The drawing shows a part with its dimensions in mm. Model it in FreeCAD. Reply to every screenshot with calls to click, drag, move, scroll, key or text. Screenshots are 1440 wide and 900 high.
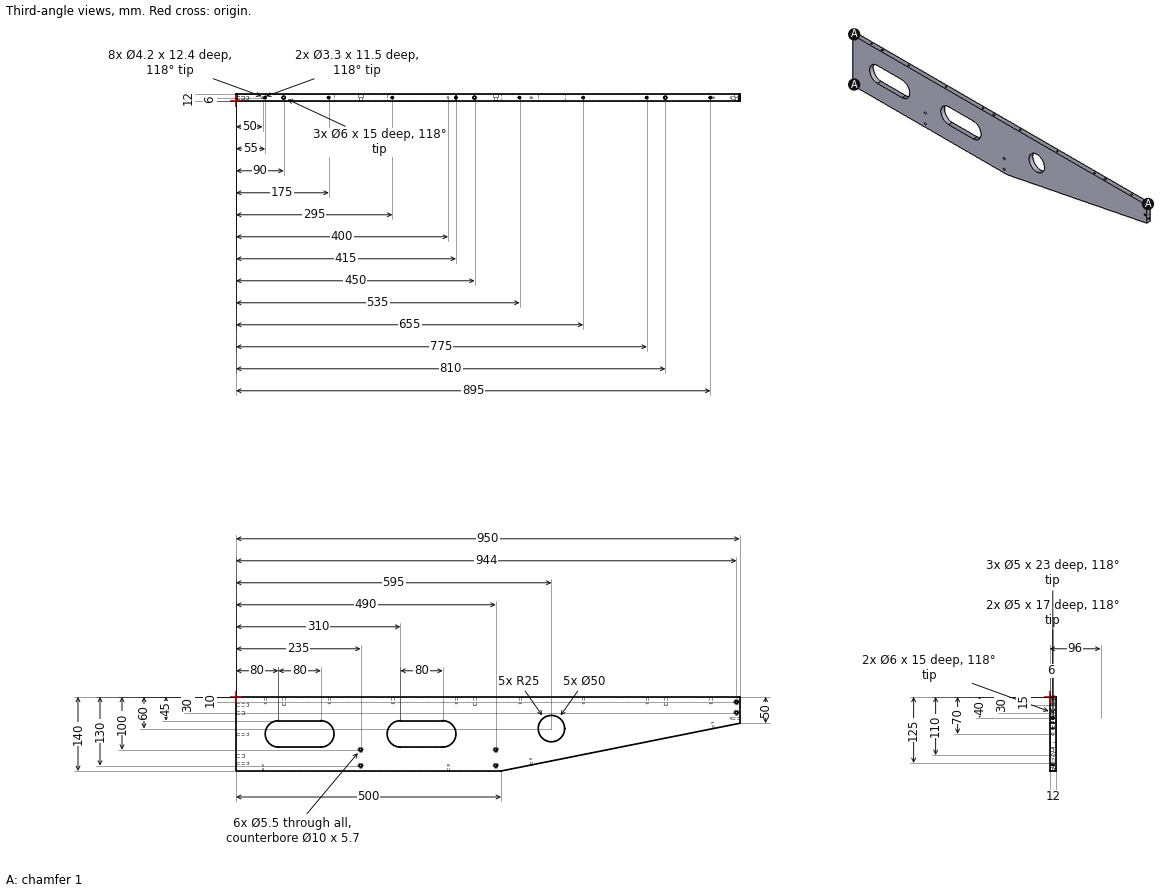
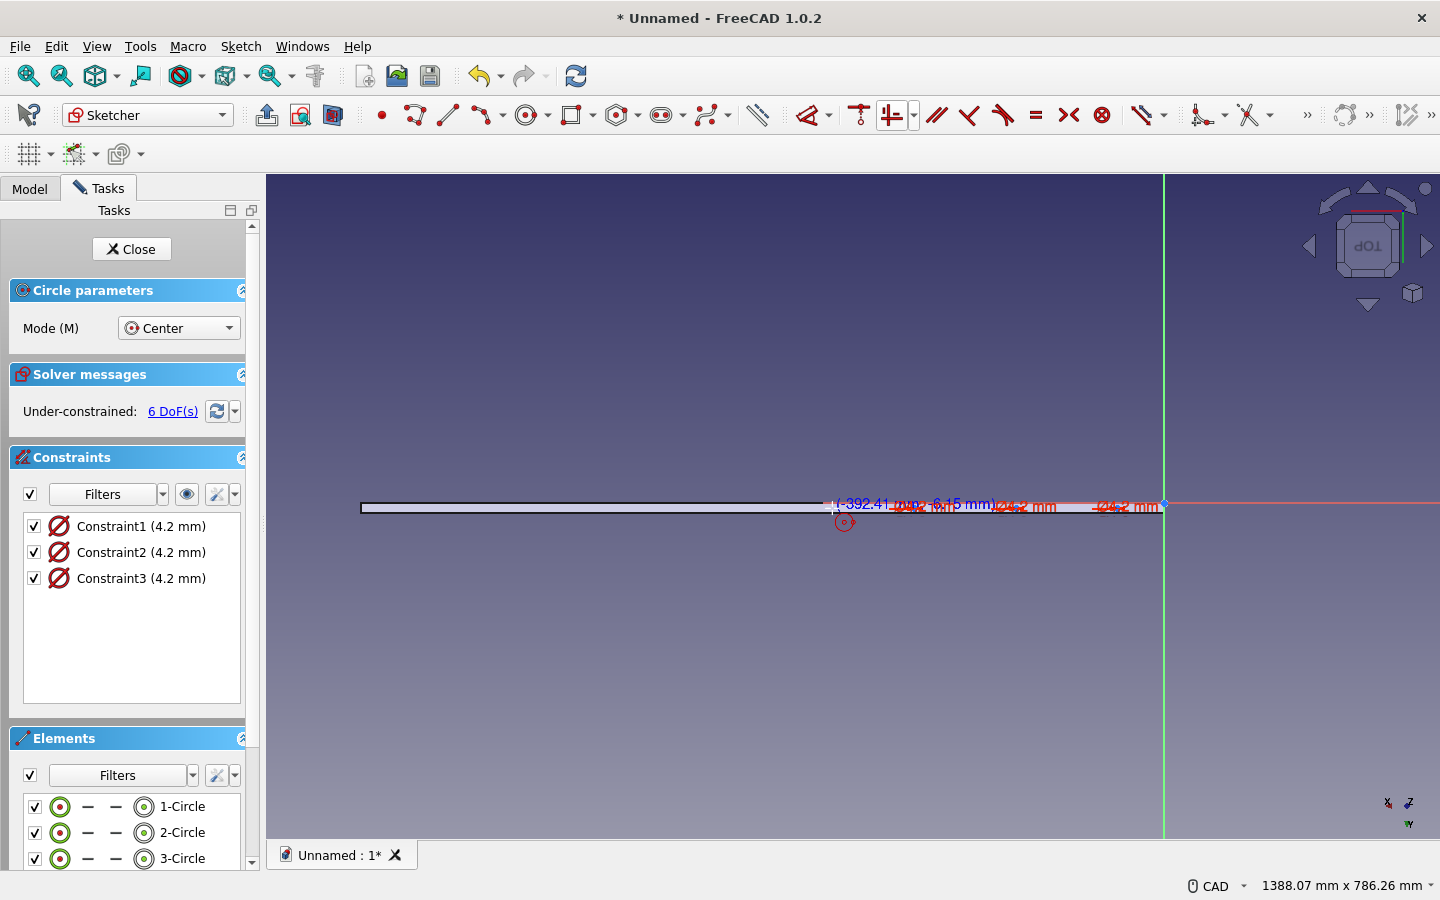
scroll(813, 508, up, 6)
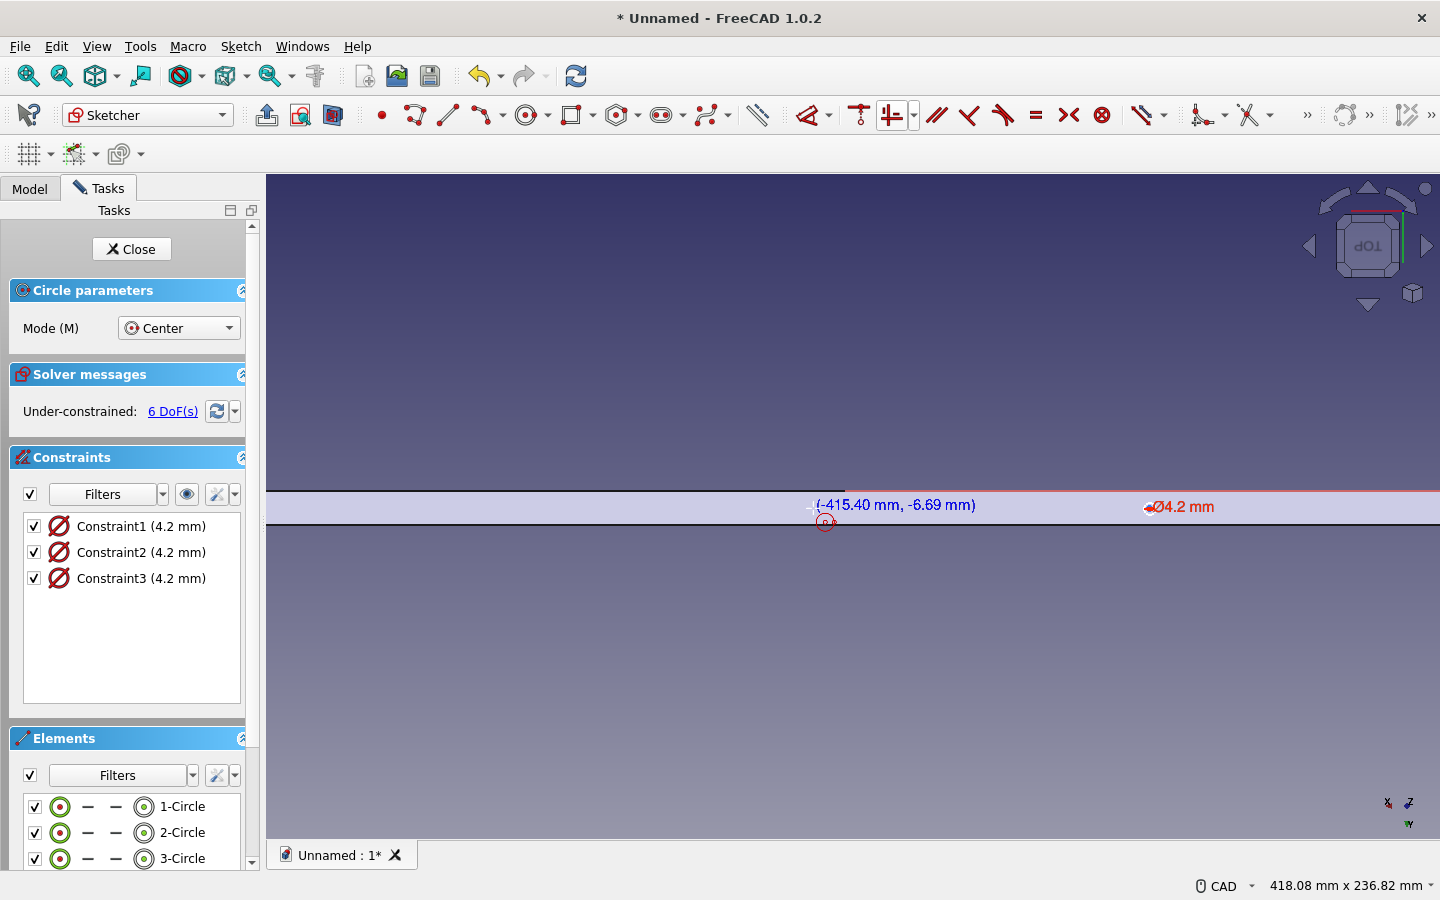
click(813, 508)
move(817, 512)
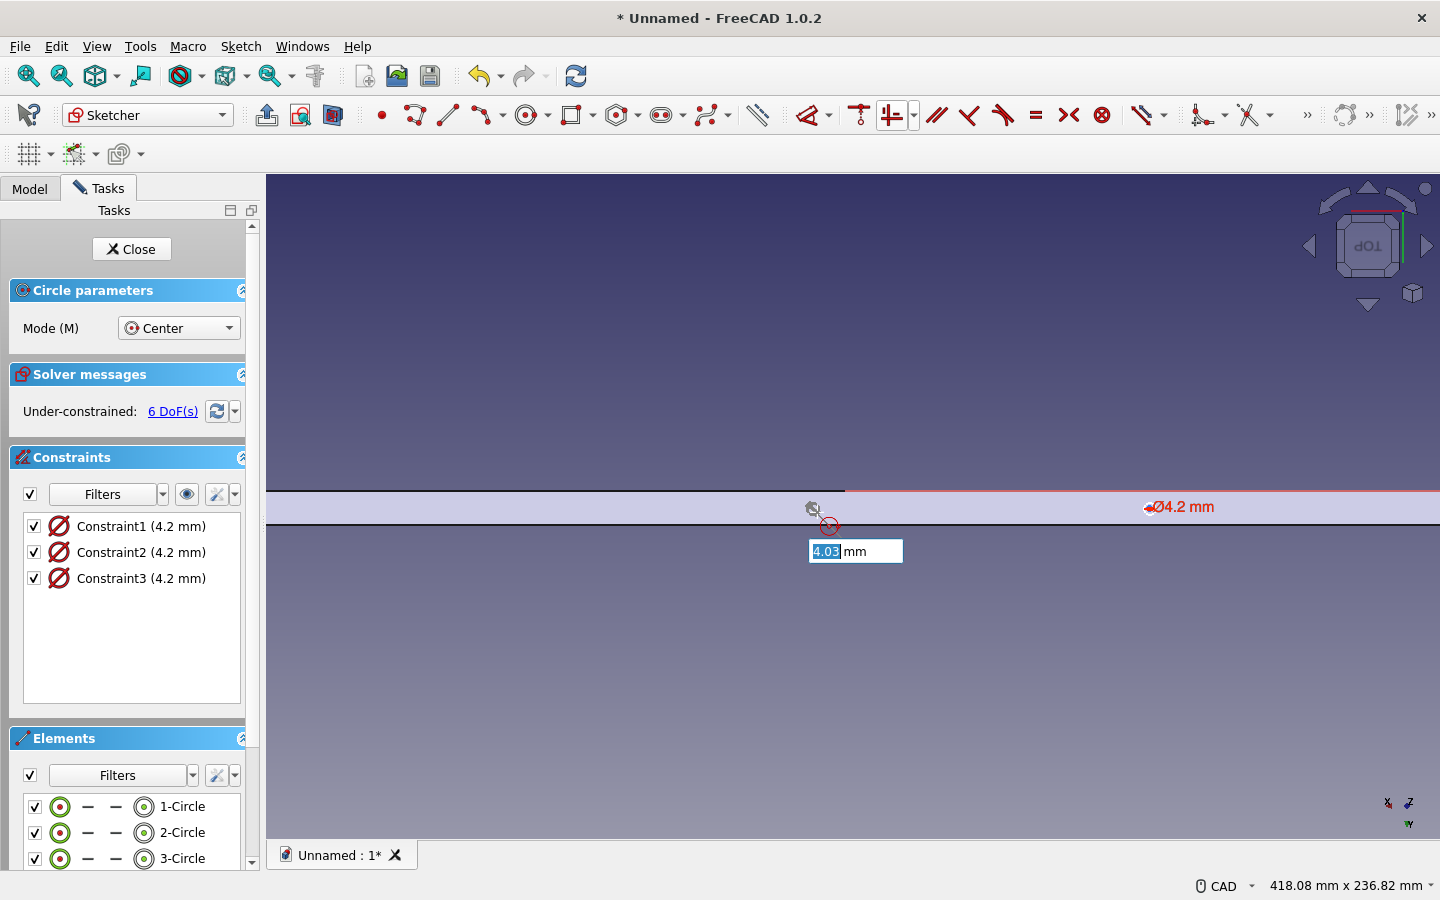
text(4.2)
key(Return)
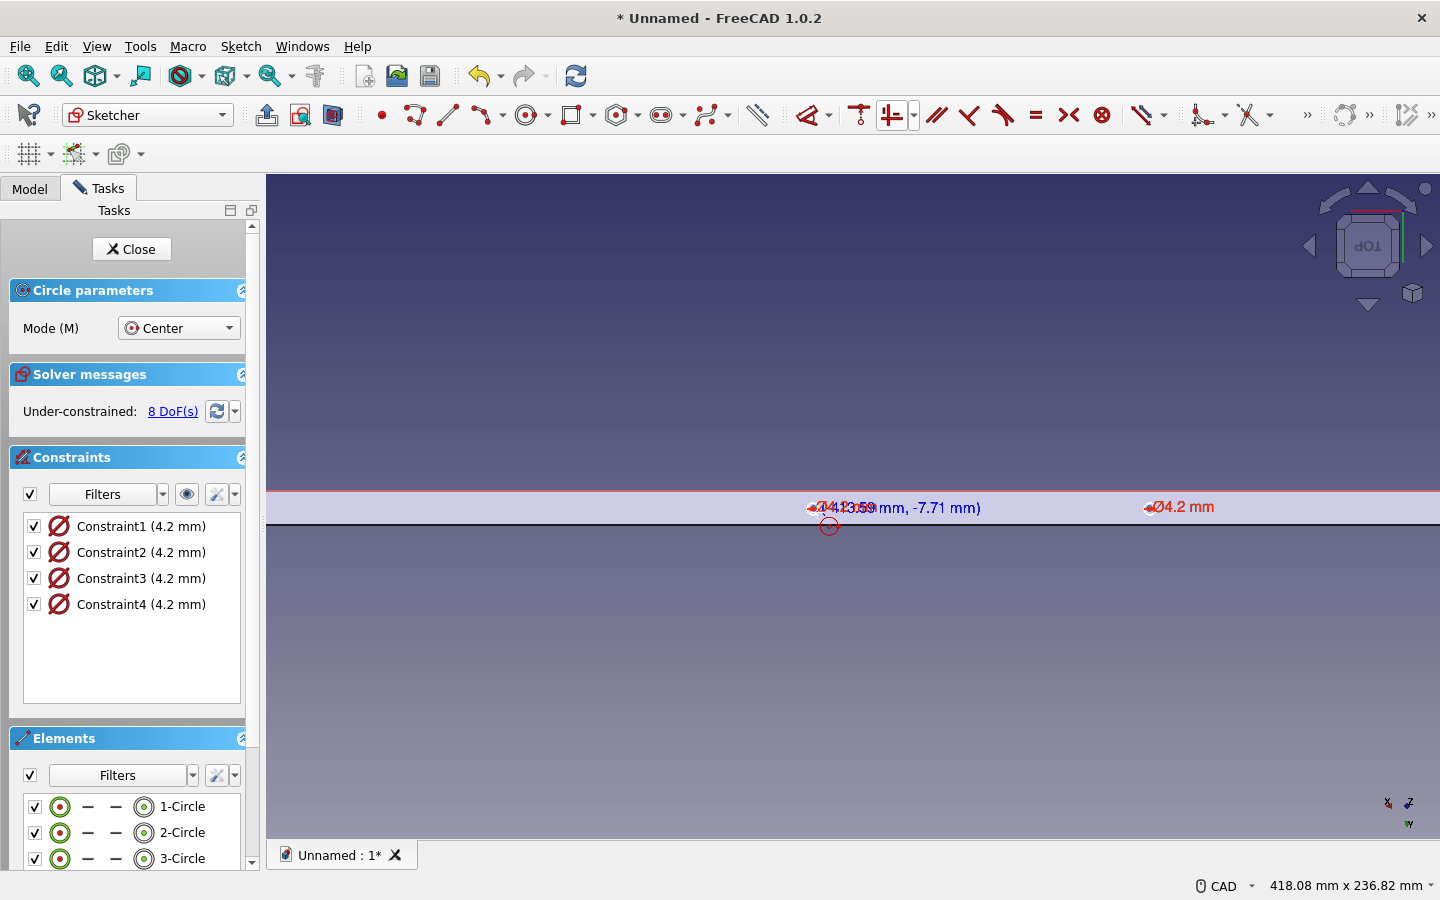
scroll(476, 508, up, 7)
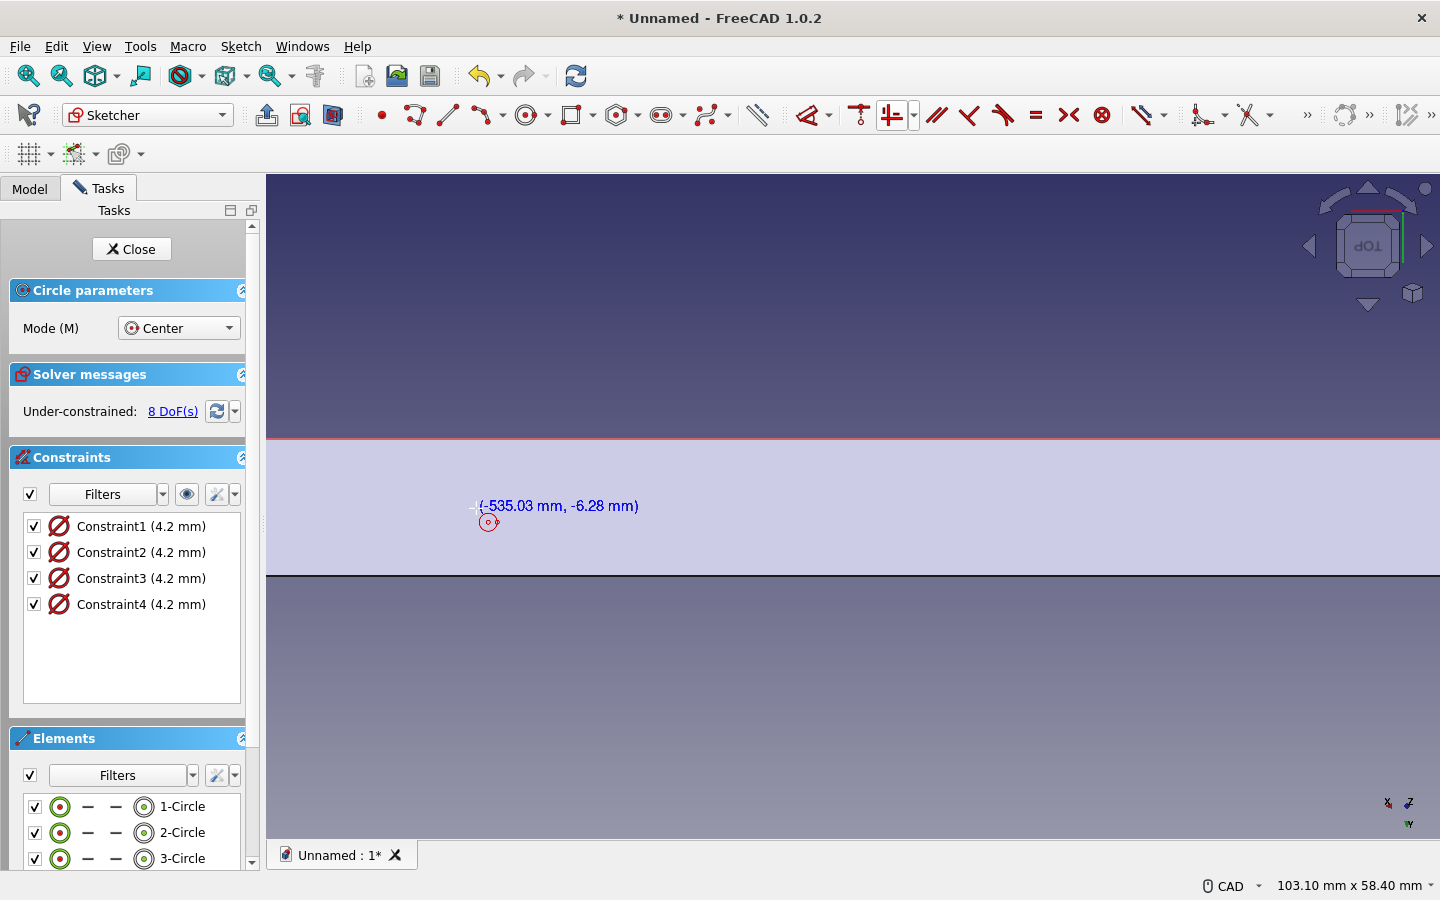
scroll(730, 508, down, 13)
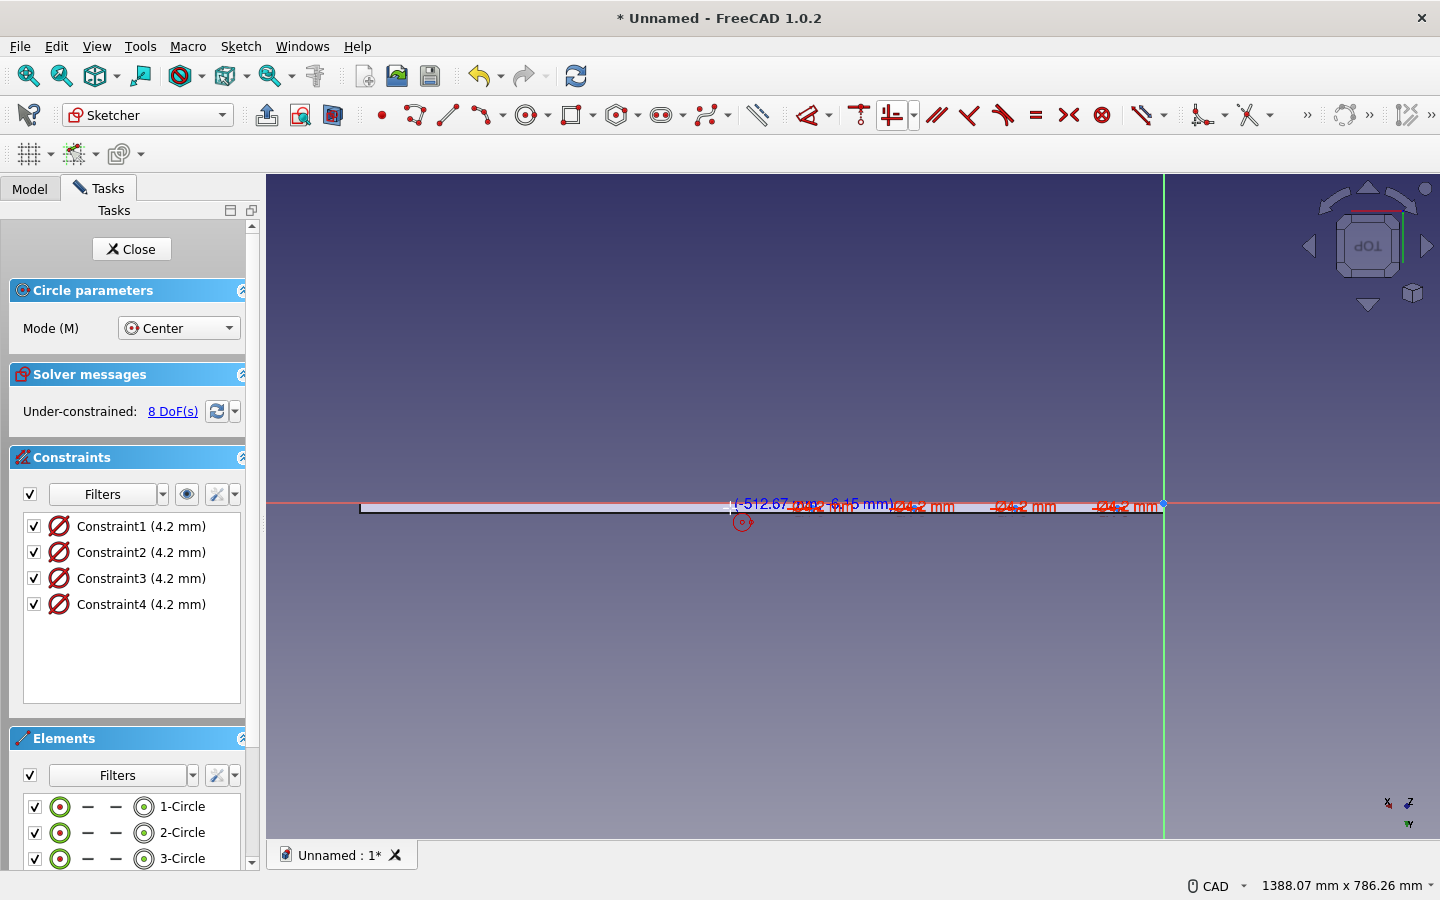
scroll(711, 508, up, 6)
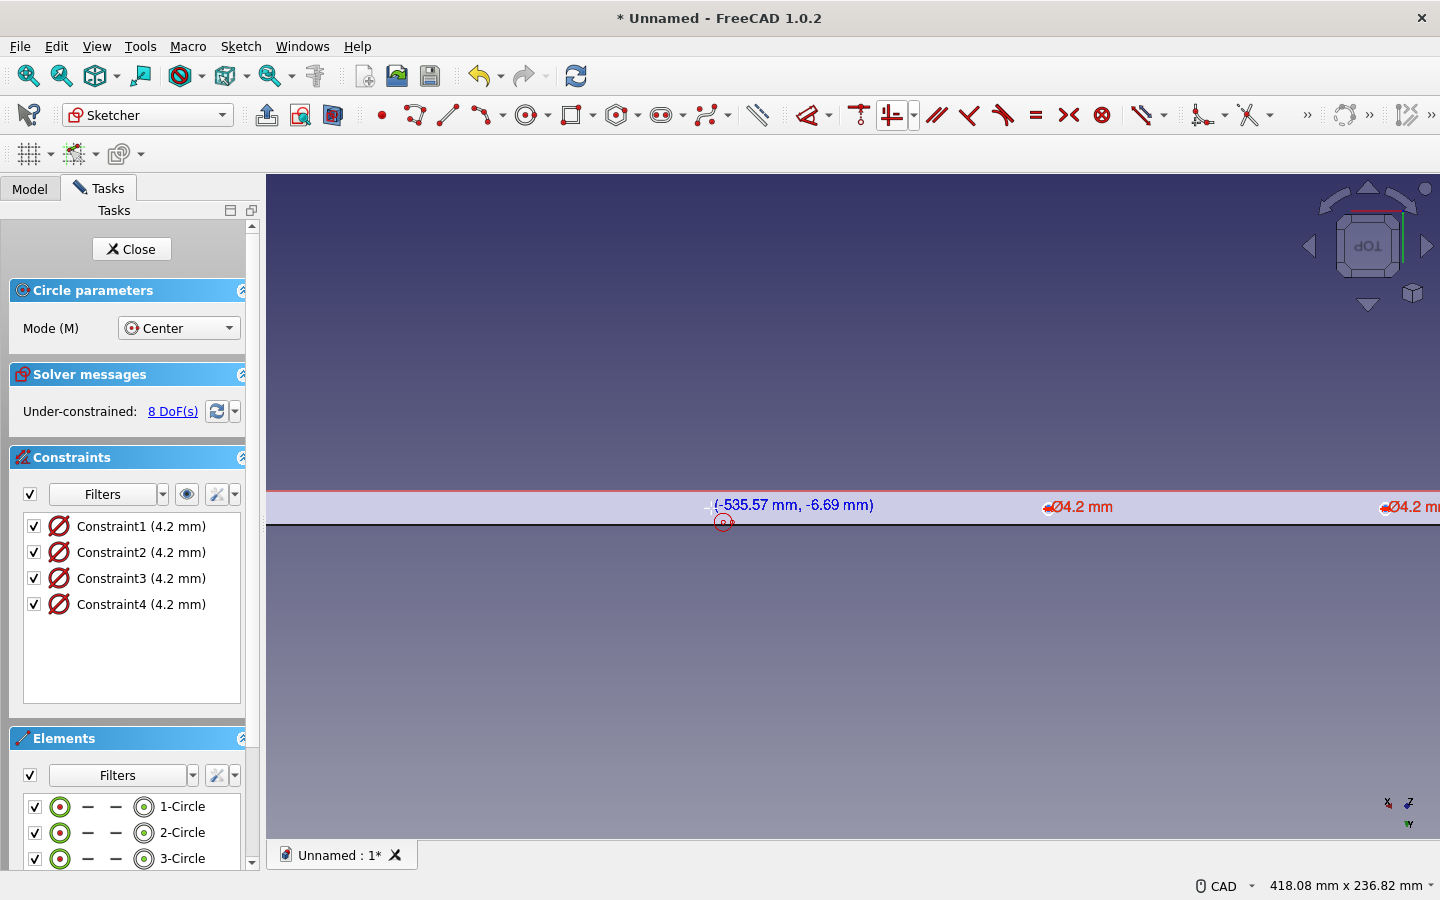
click(712, 508)
move(716, 512)